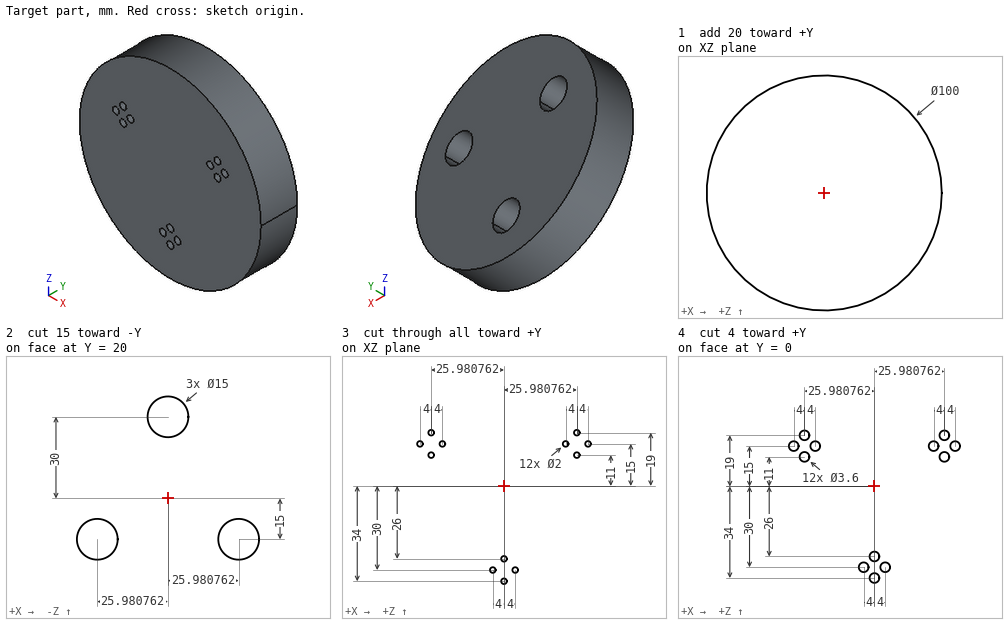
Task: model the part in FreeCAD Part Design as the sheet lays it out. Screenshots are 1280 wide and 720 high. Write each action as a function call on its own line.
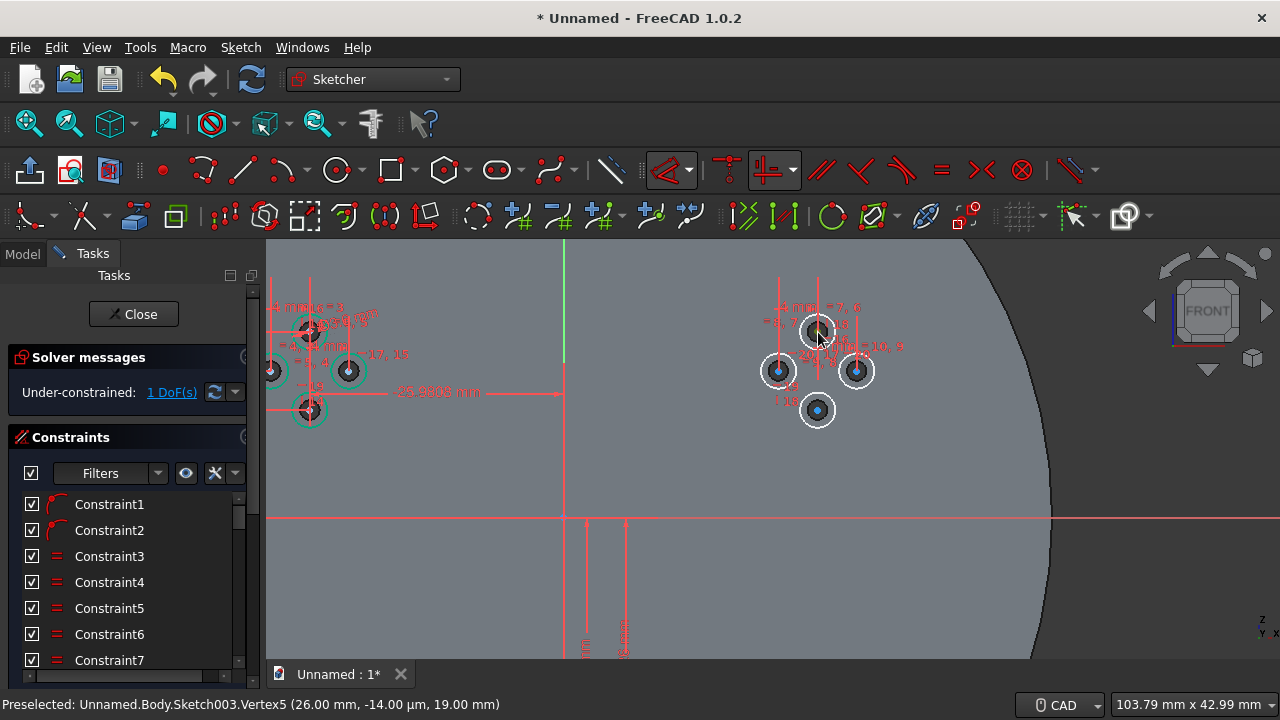
click(692, 170)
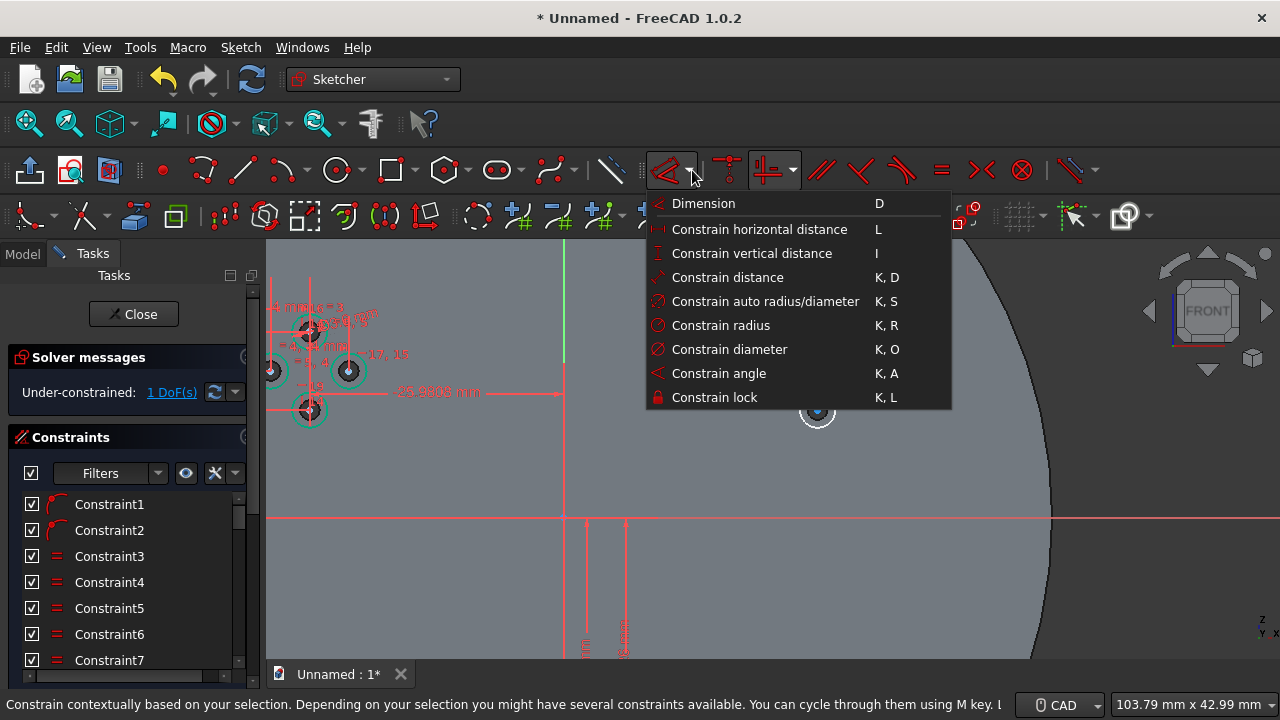
click(799, 229)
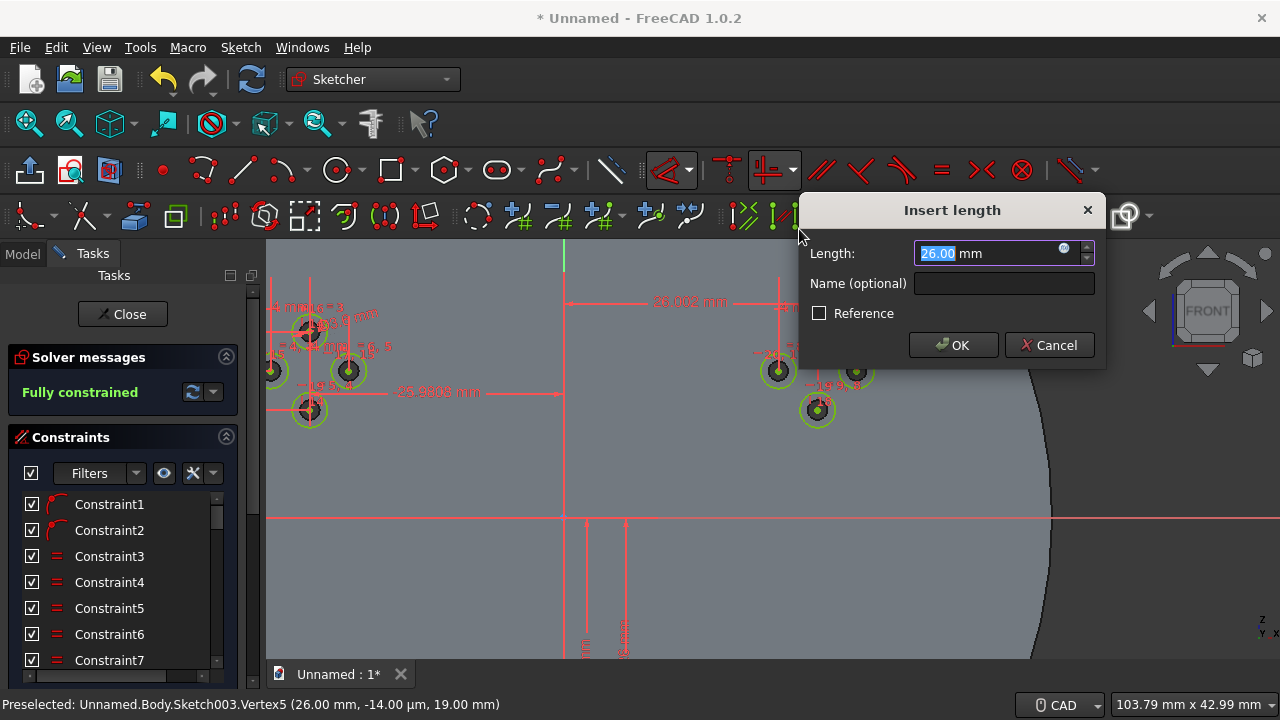
text(25.980762)
key(Return)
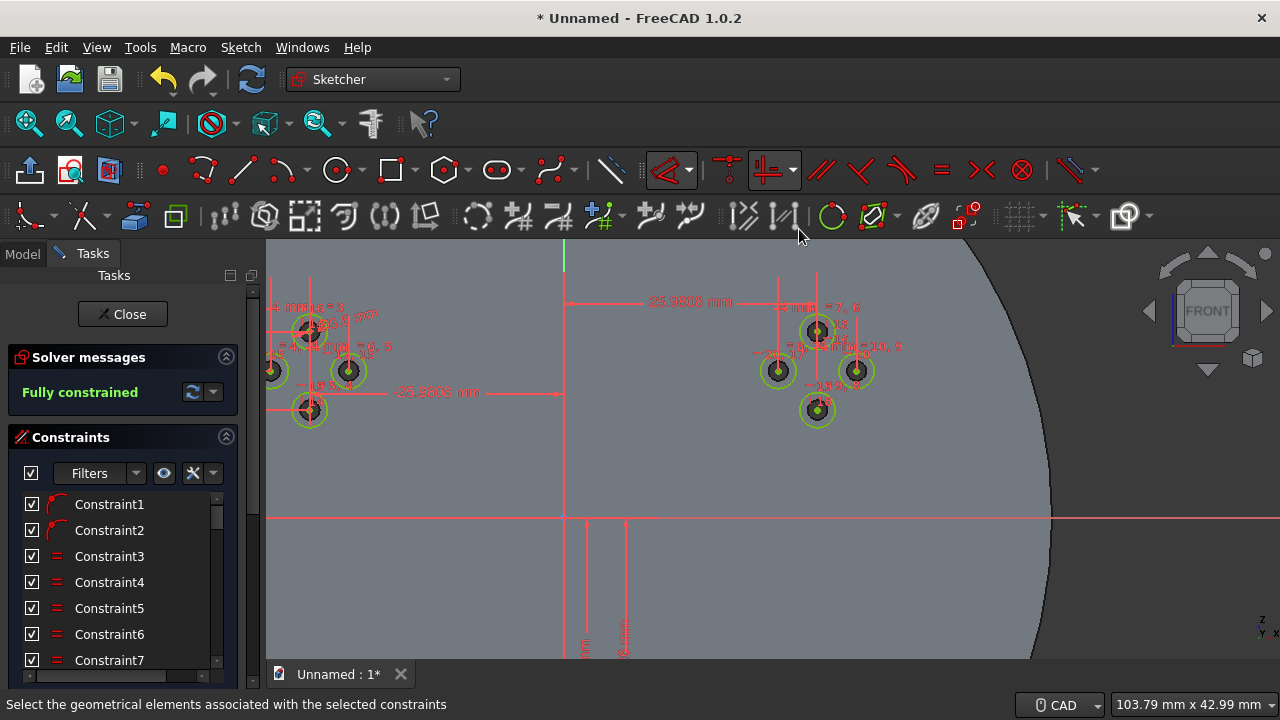
click(123, 314)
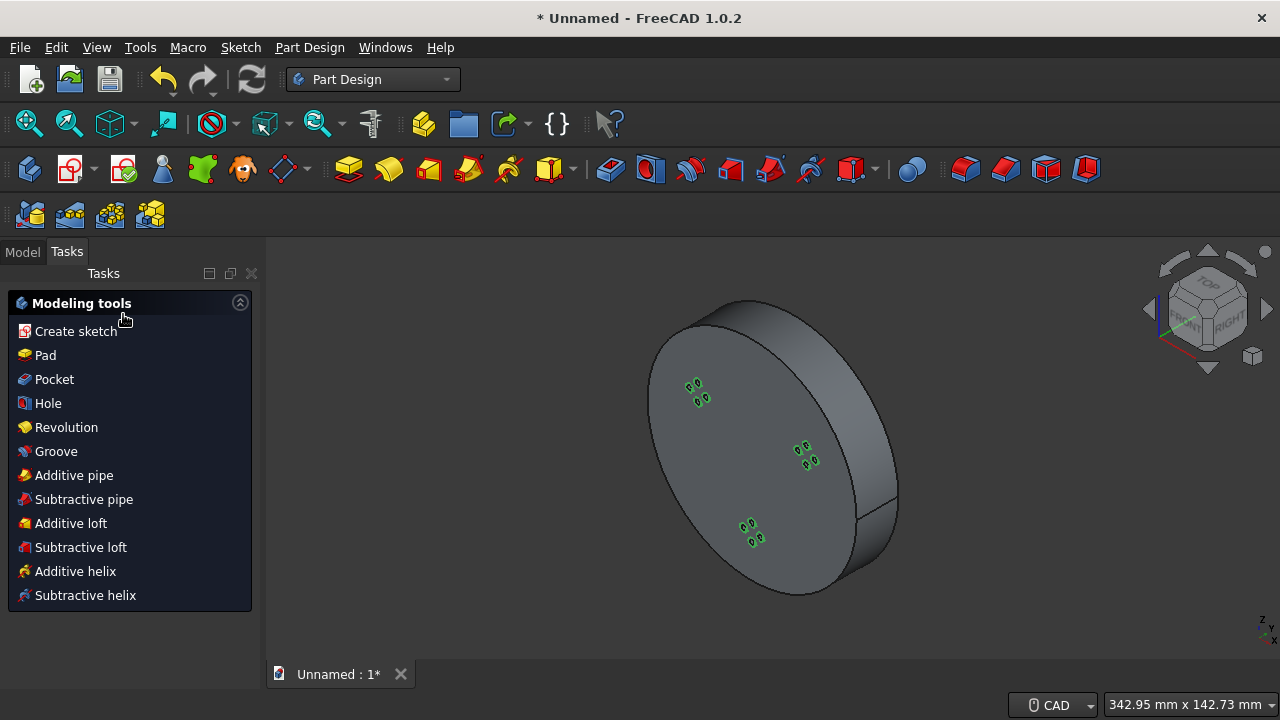
click(612, 170)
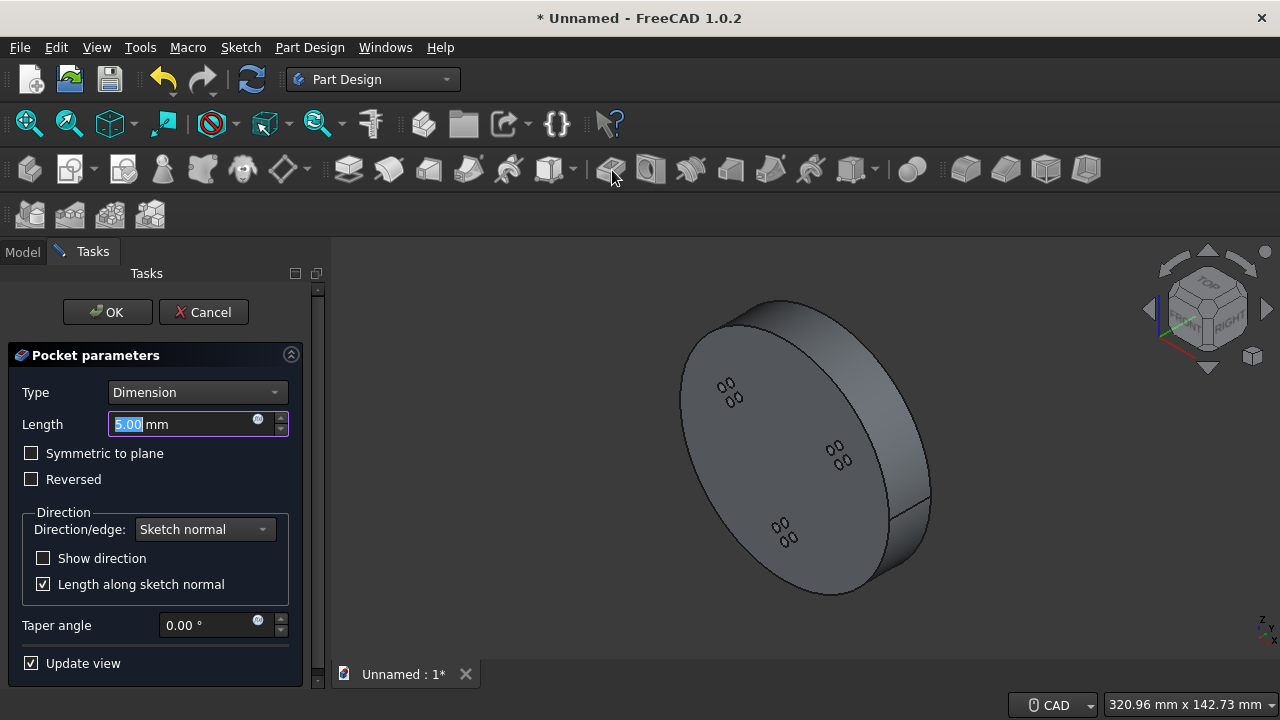
text(4)
key(Tab)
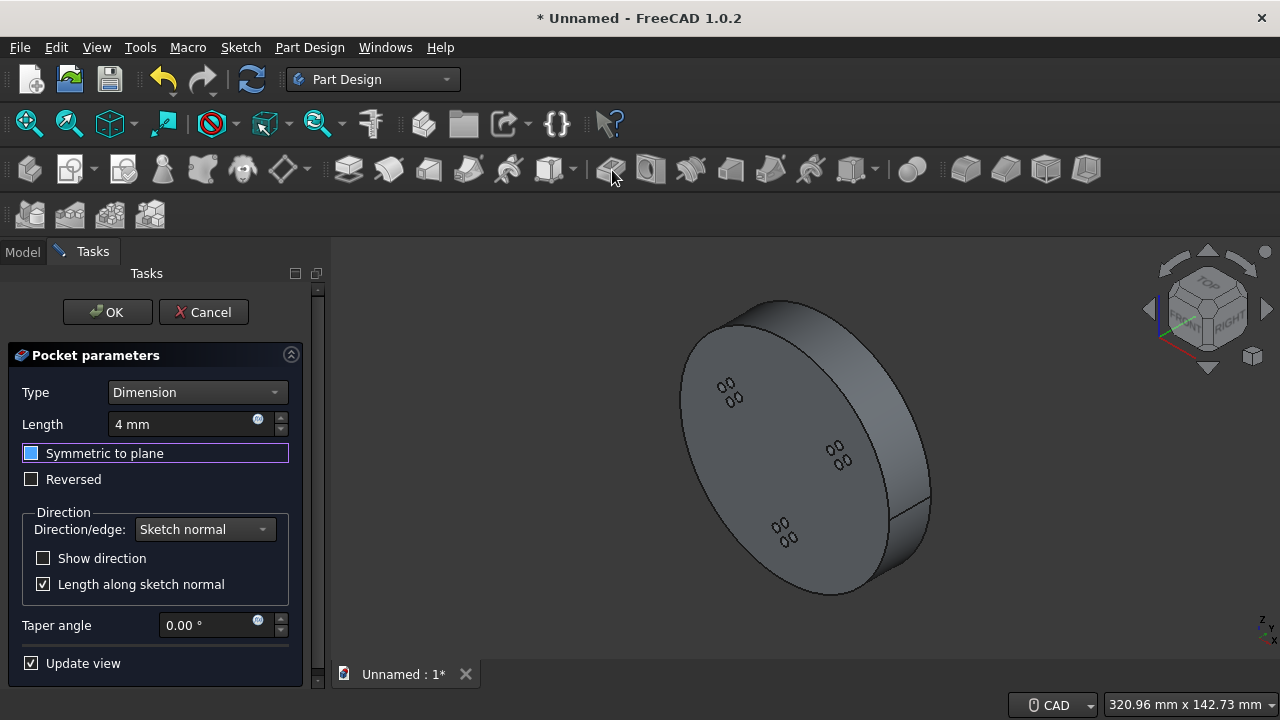
click(108, 312)